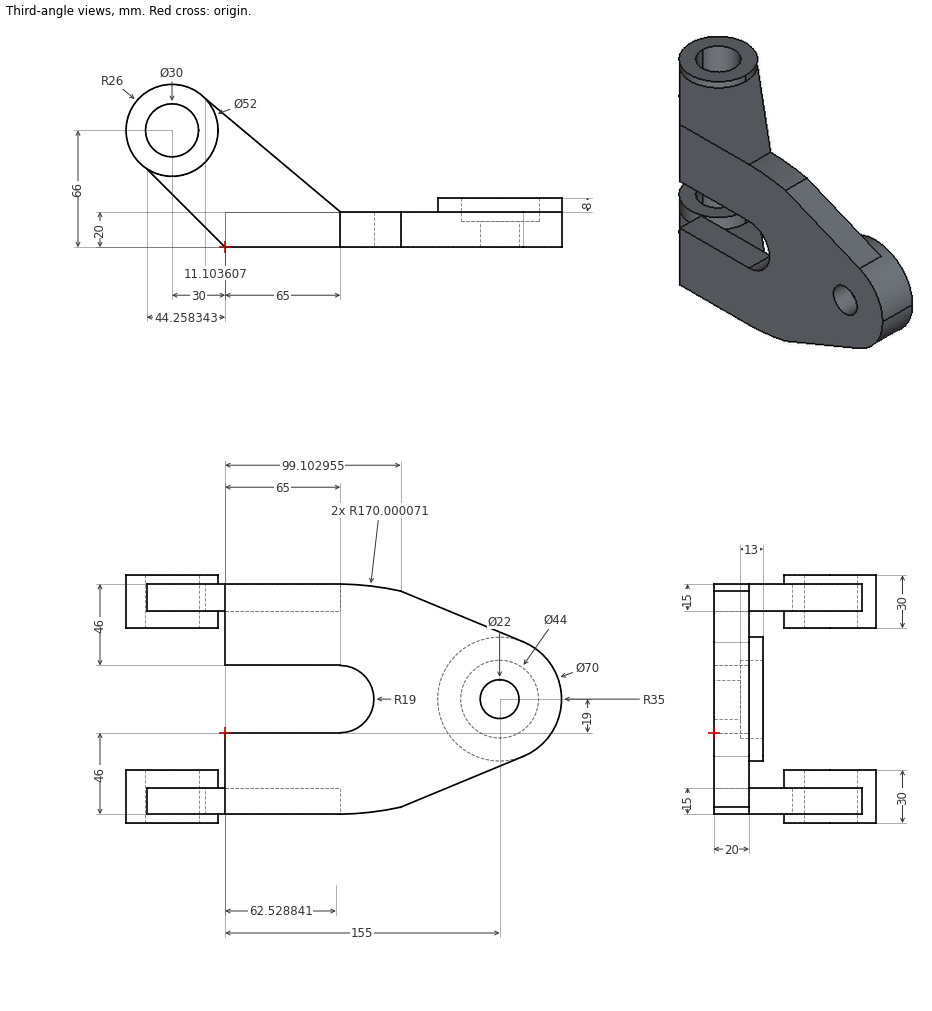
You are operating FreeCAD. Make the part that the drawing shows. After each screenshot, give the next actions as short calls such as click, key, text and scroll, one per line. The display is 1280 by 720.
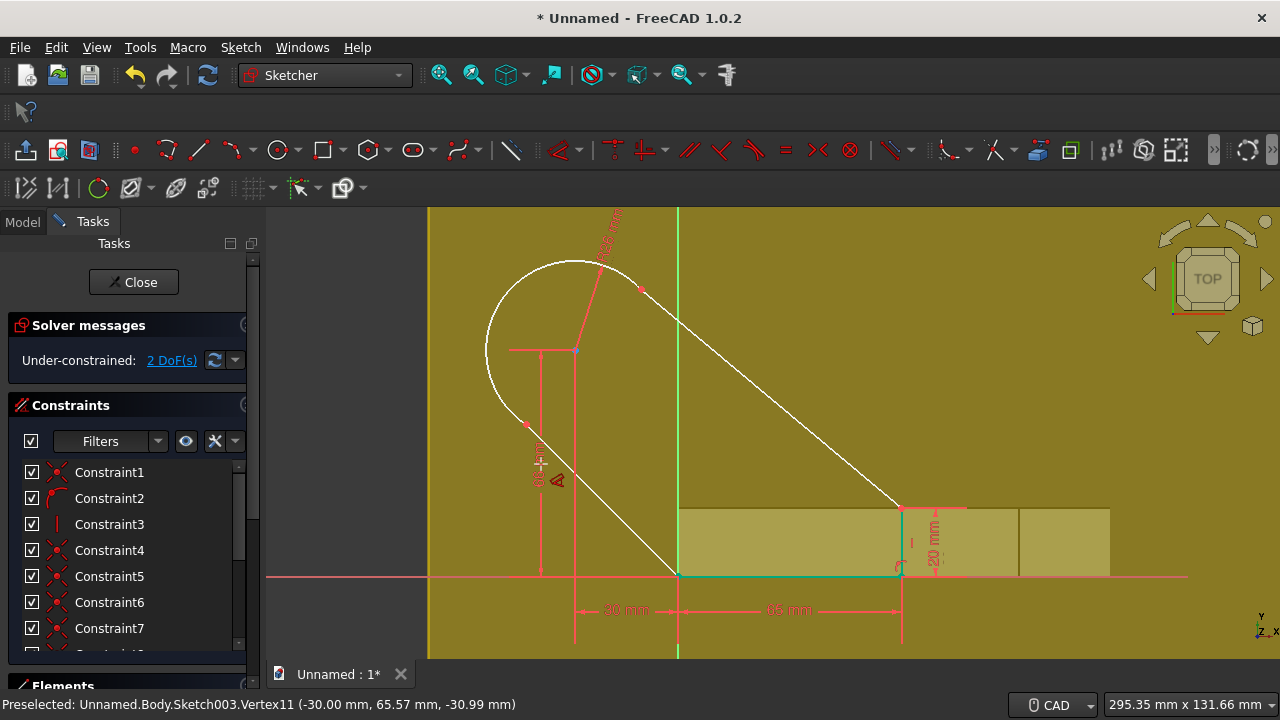
click(641, 290)
click(660, 256)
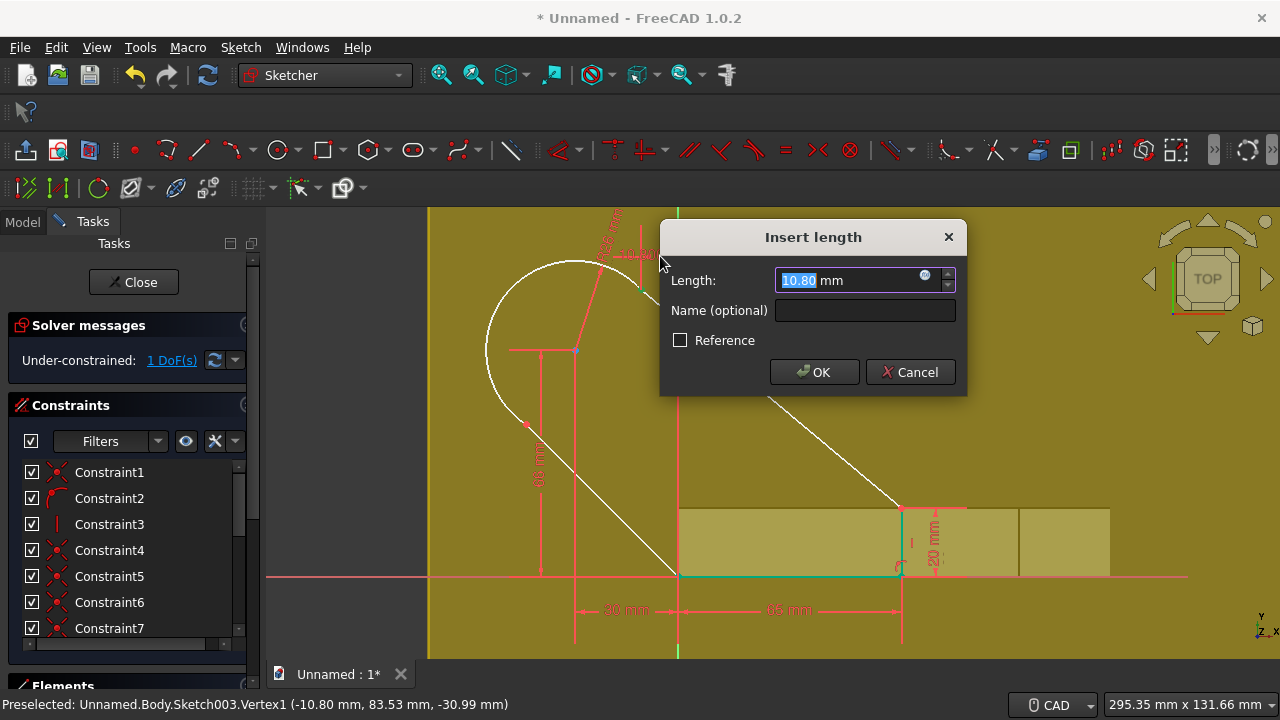
text(11.103607)
key(Return)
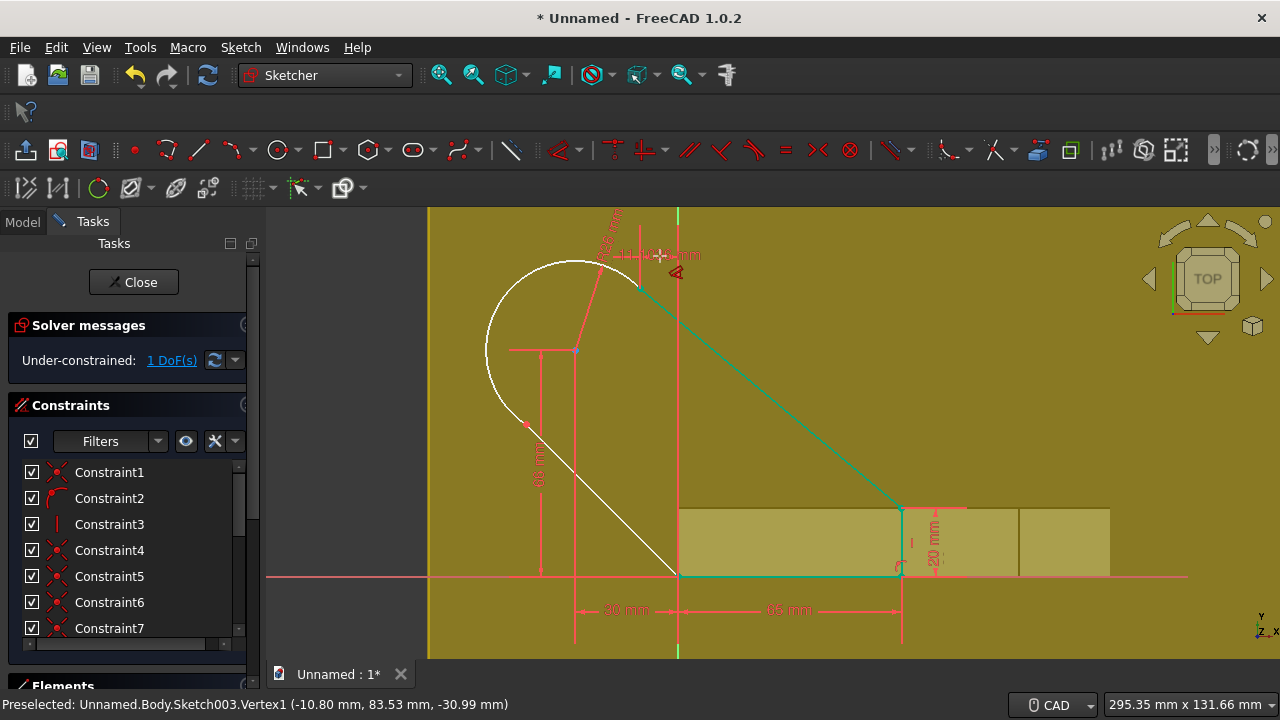
click(526, 425)
click(549, 611)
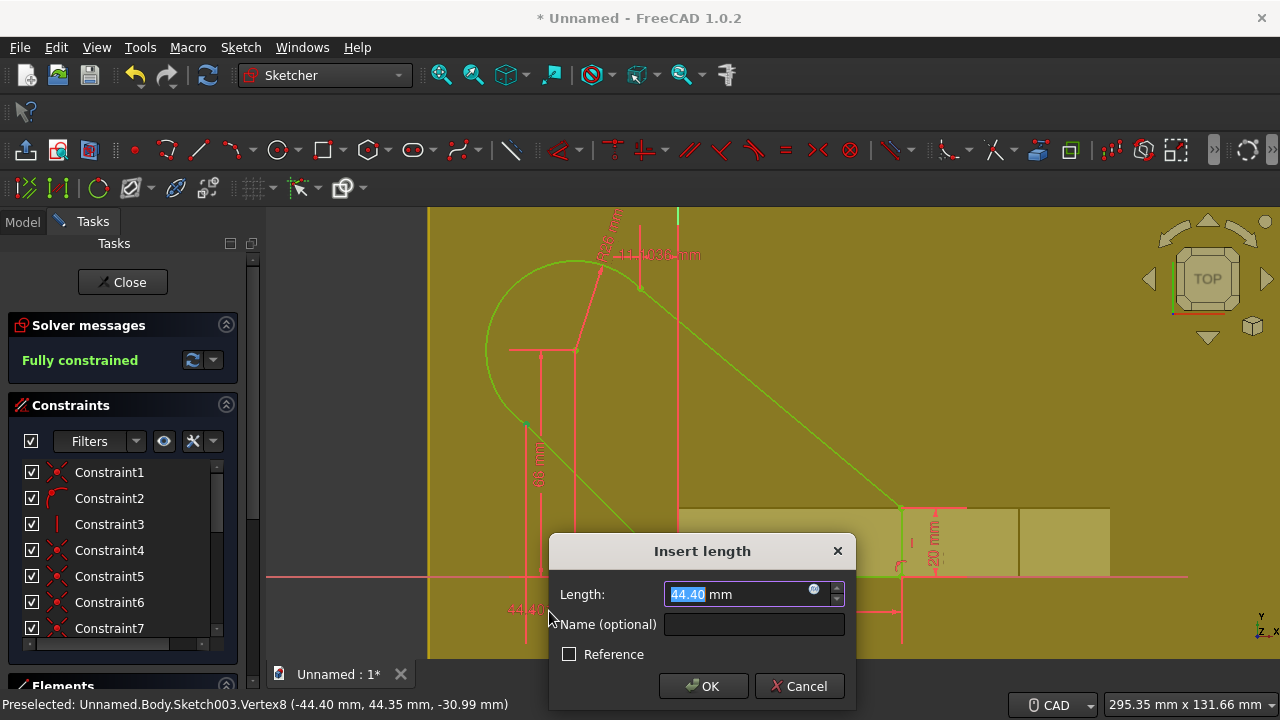
text(44.258343)
key(Return)
key(Escape)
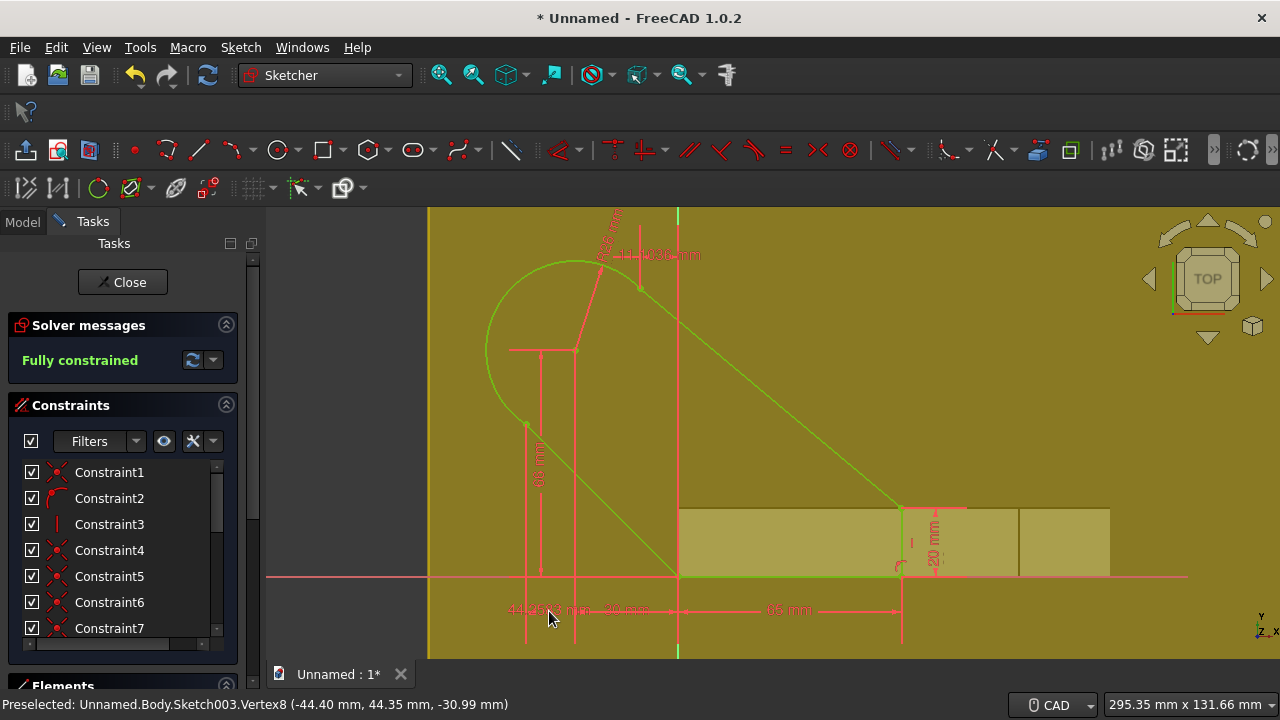
click(123, 282)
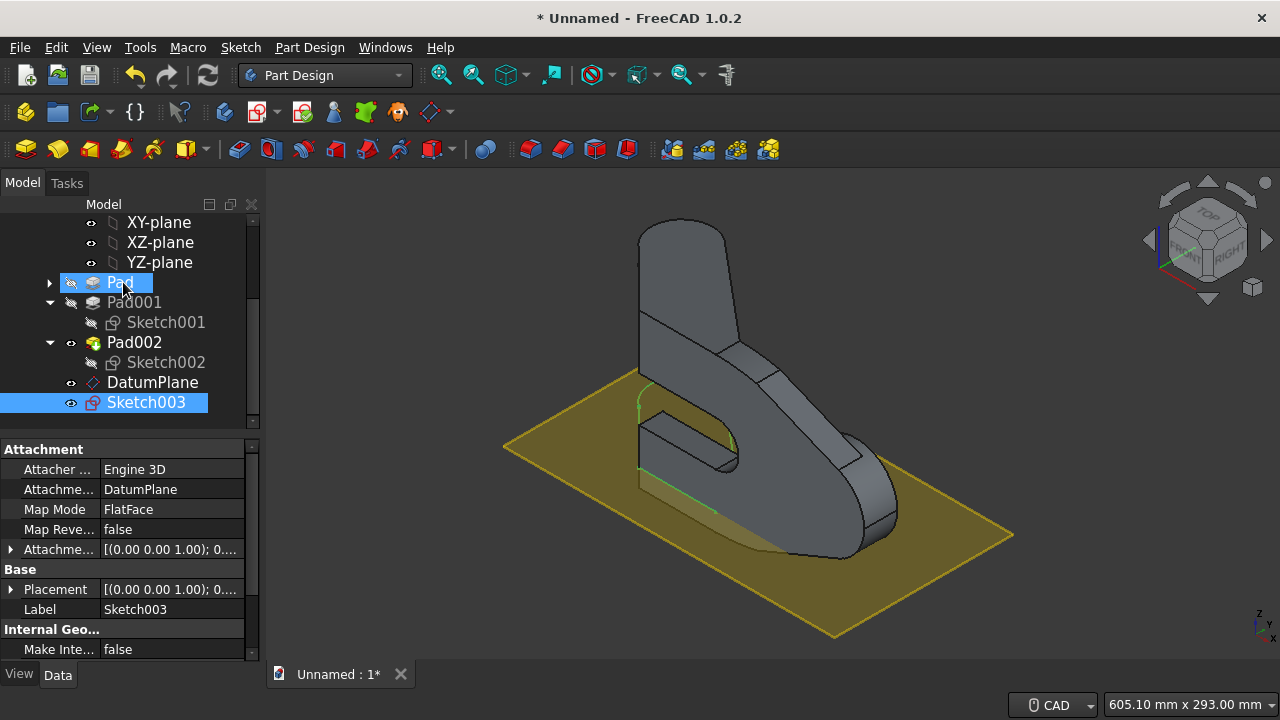
click(26, 150)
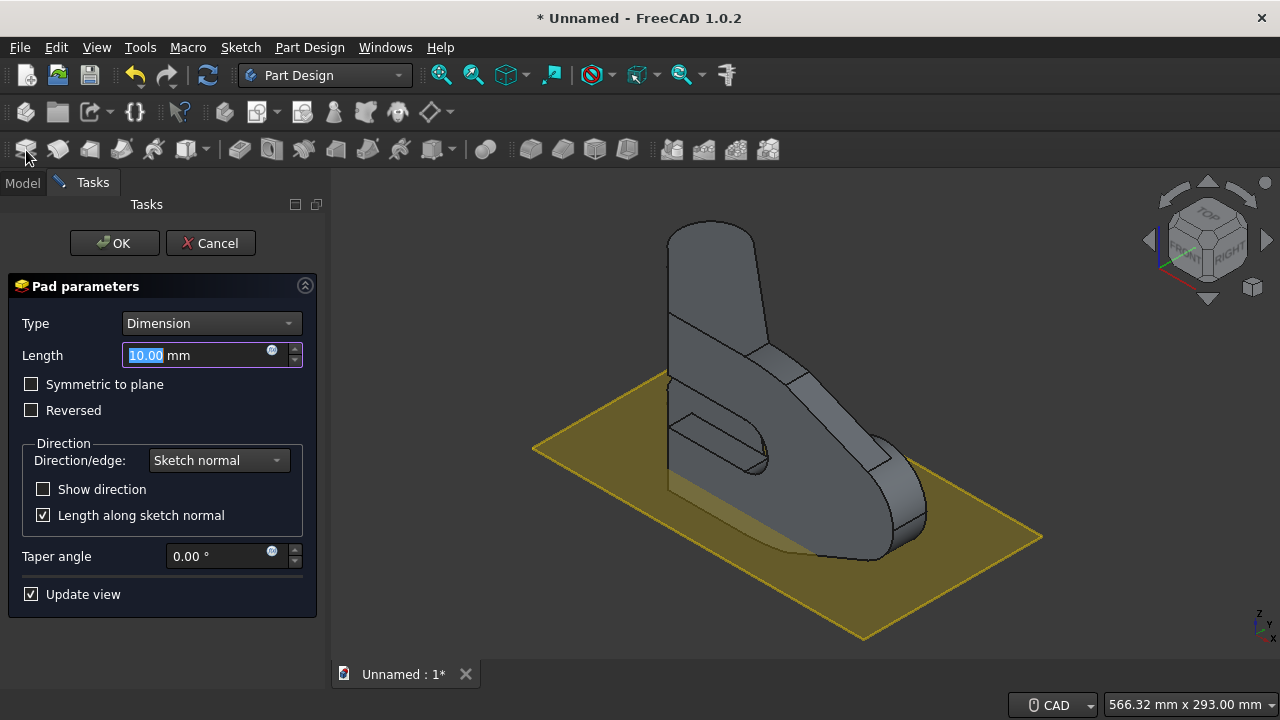
text(15)
key(Tab)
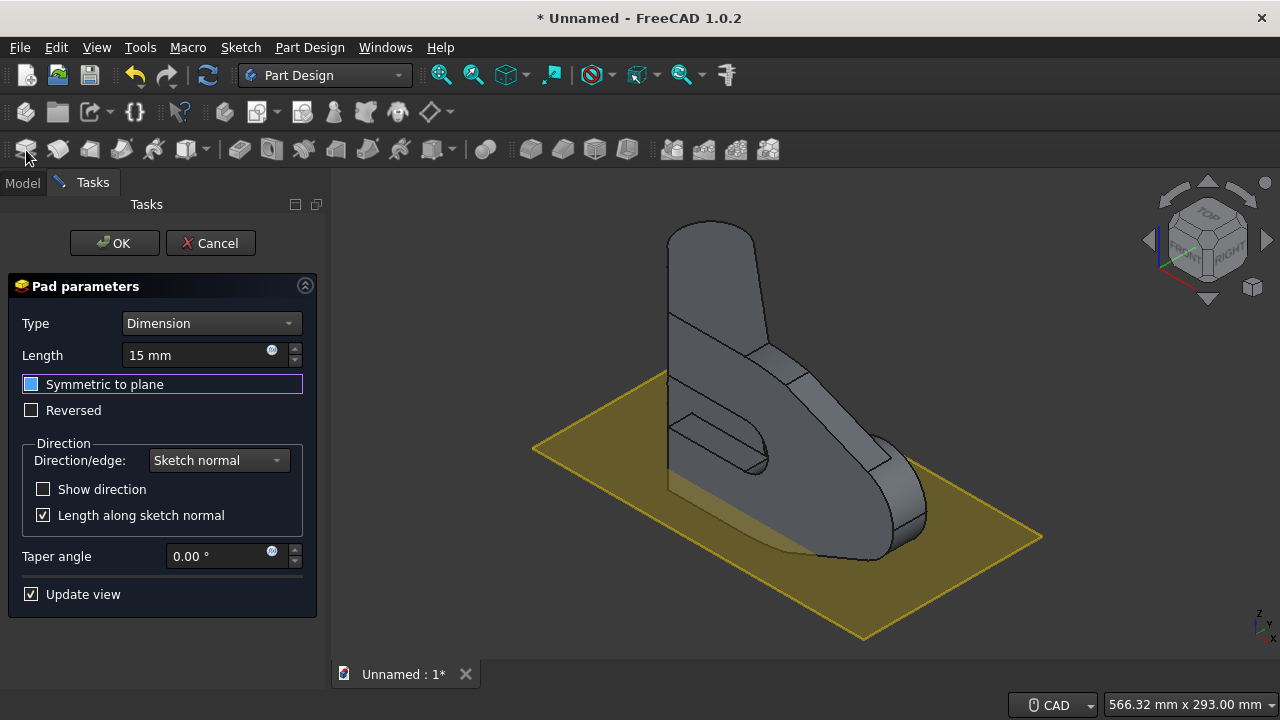
click(30, 410)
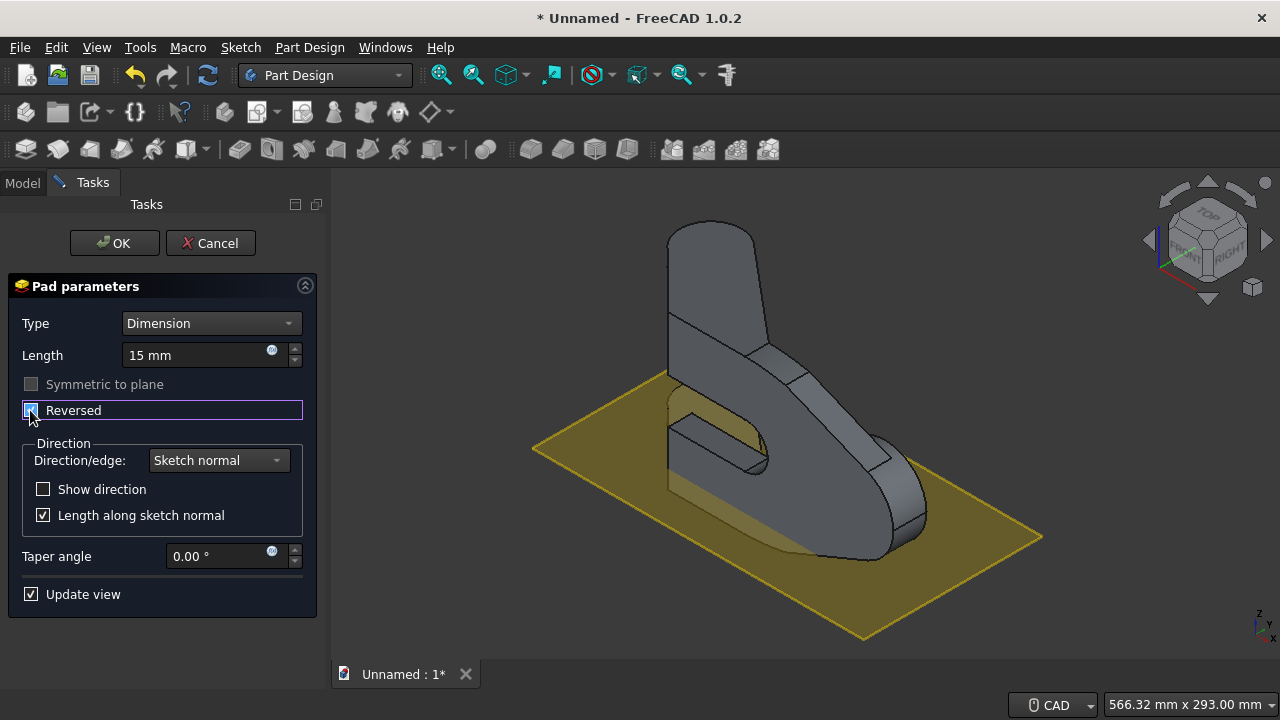
click(115, 243)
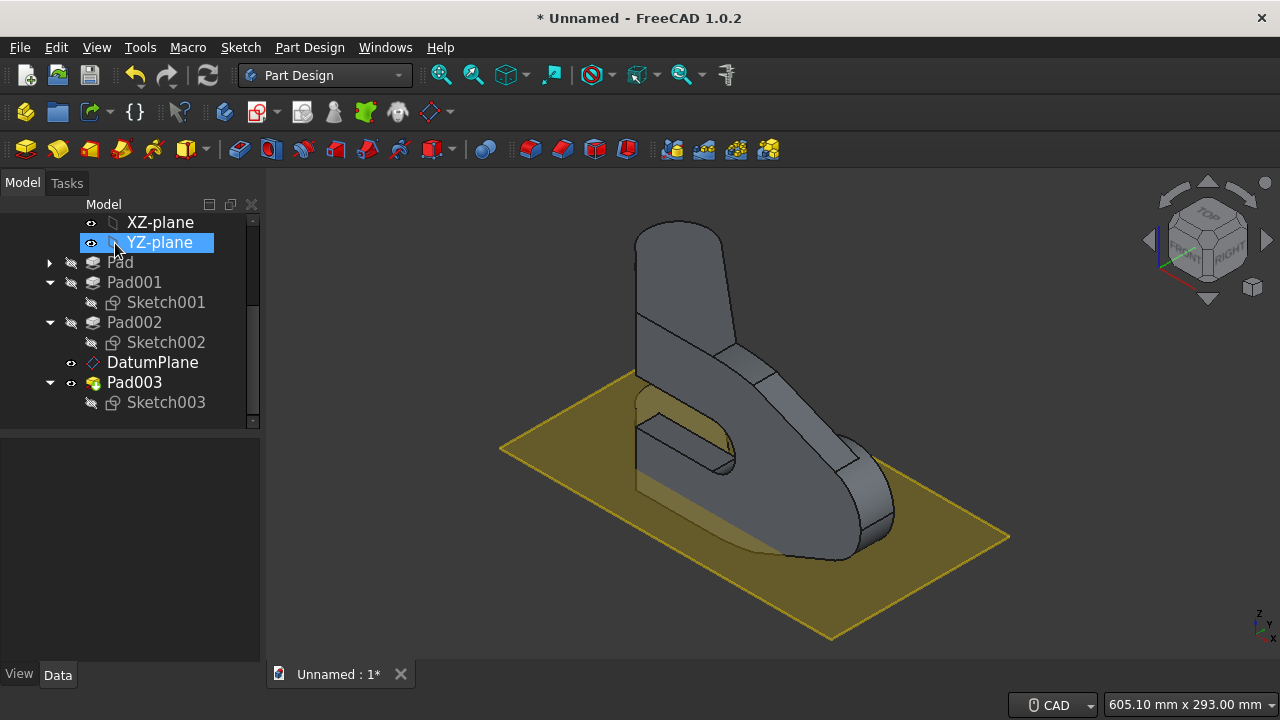
click(116, 363)
key(space)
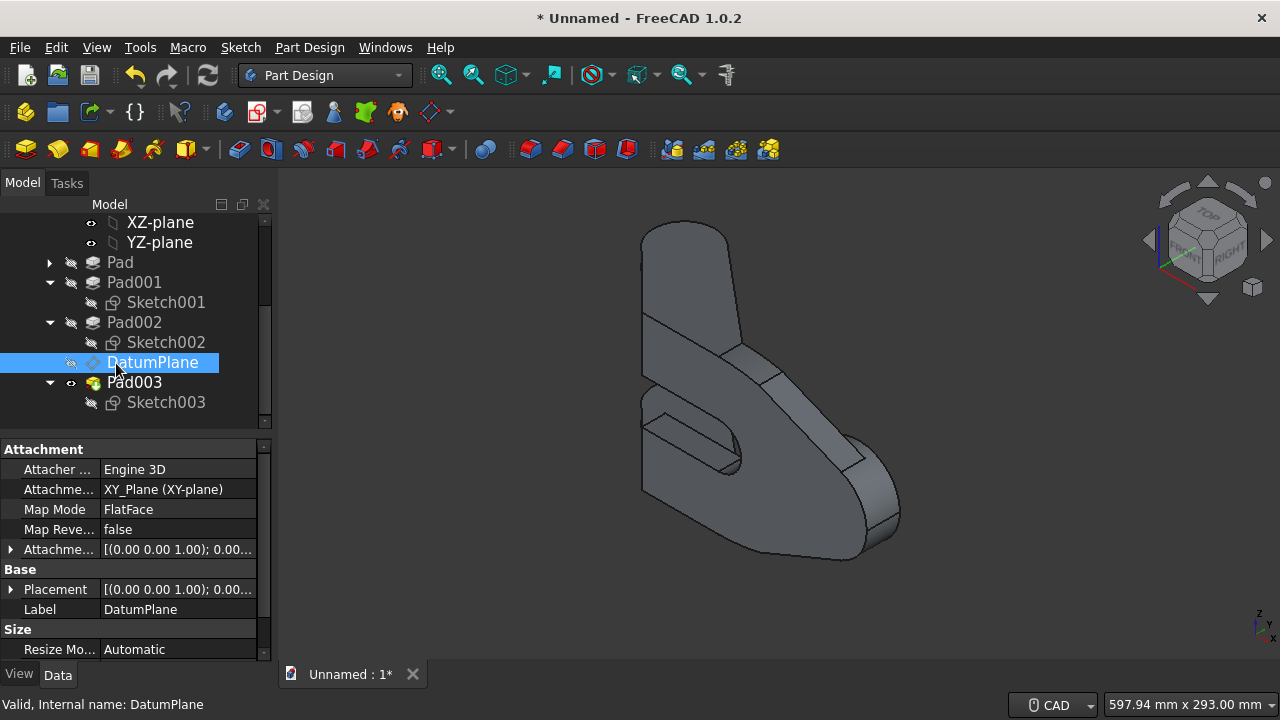
scroll(160, 318, down, 3)